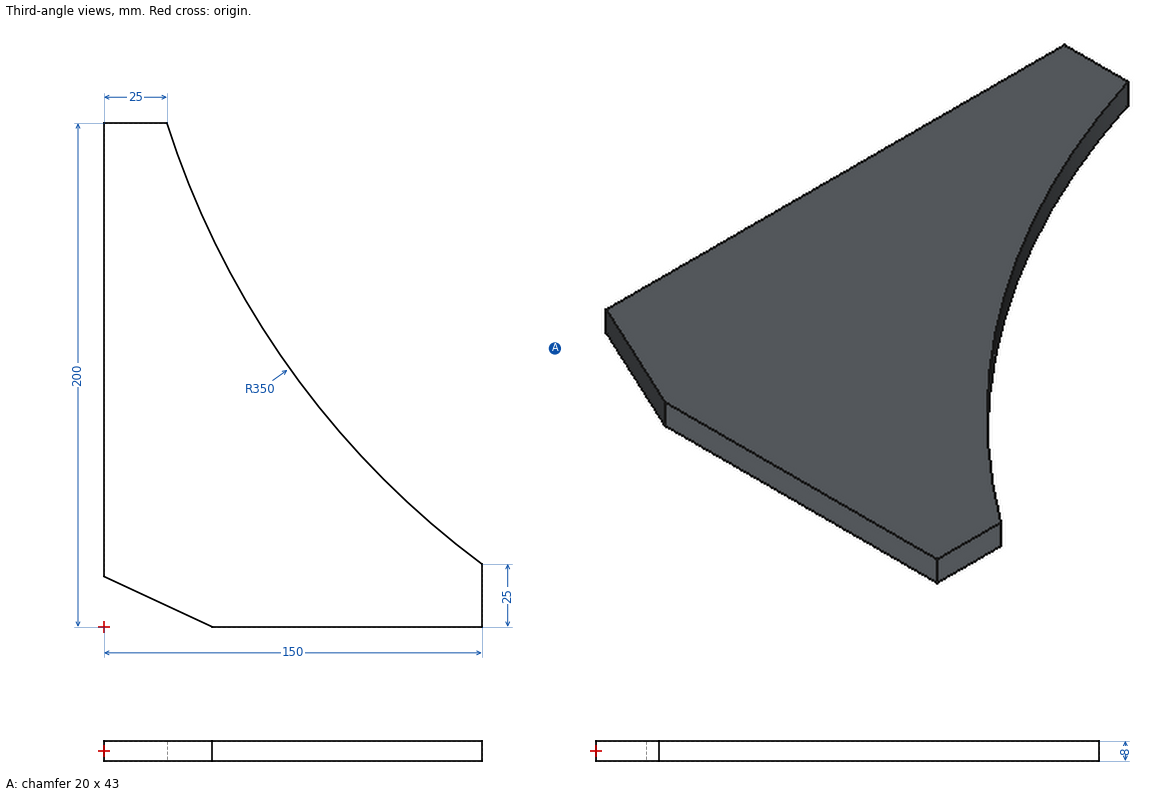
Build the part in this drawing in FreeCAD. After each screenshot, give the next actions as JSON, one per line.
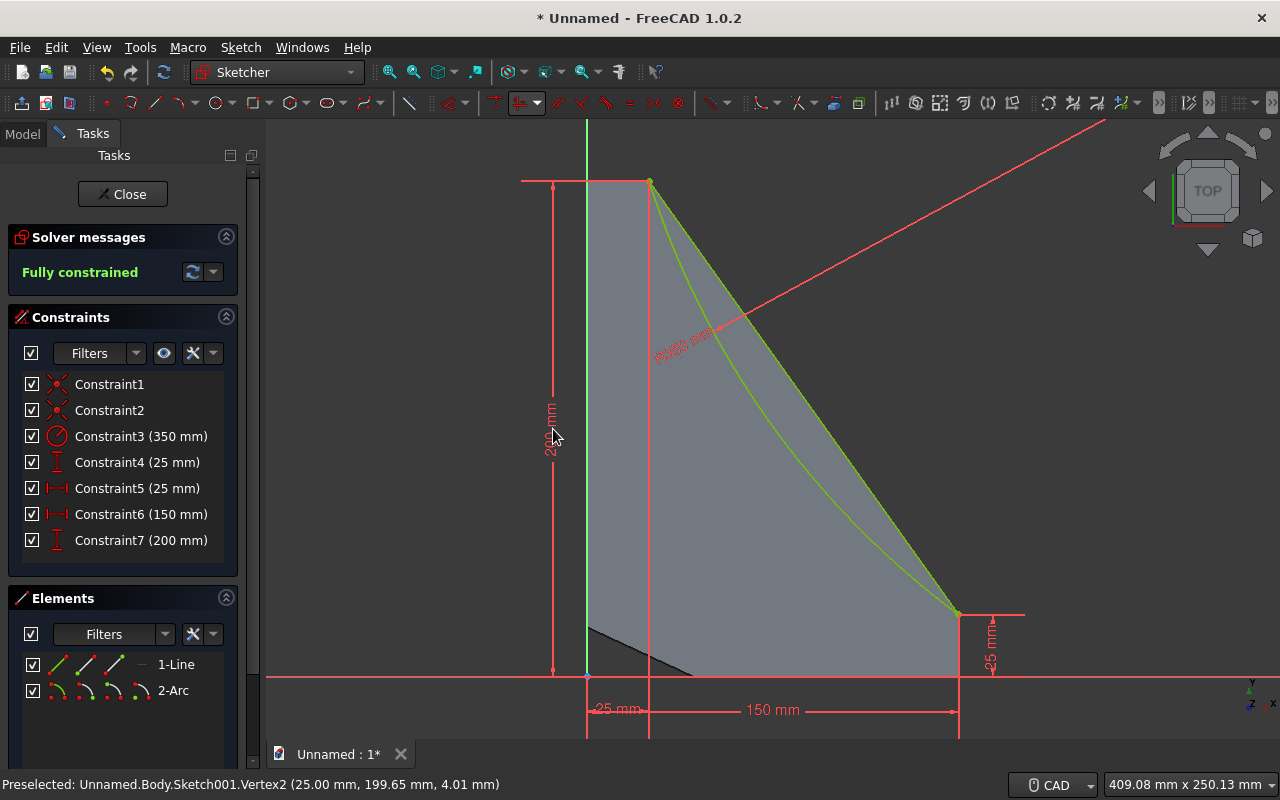
{"action": "left_click", "coordinate": [123, 194]}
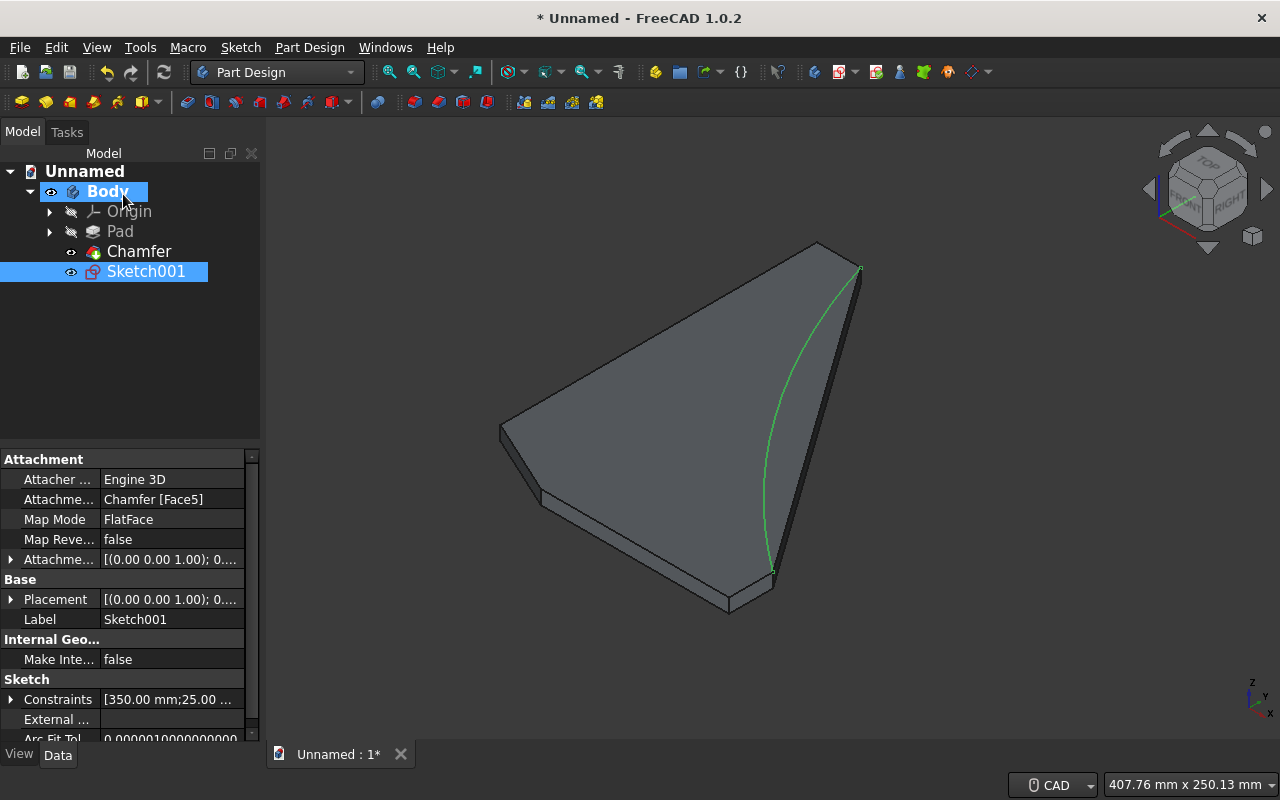
{"action": "left_click", "coordinate": [188, 102]}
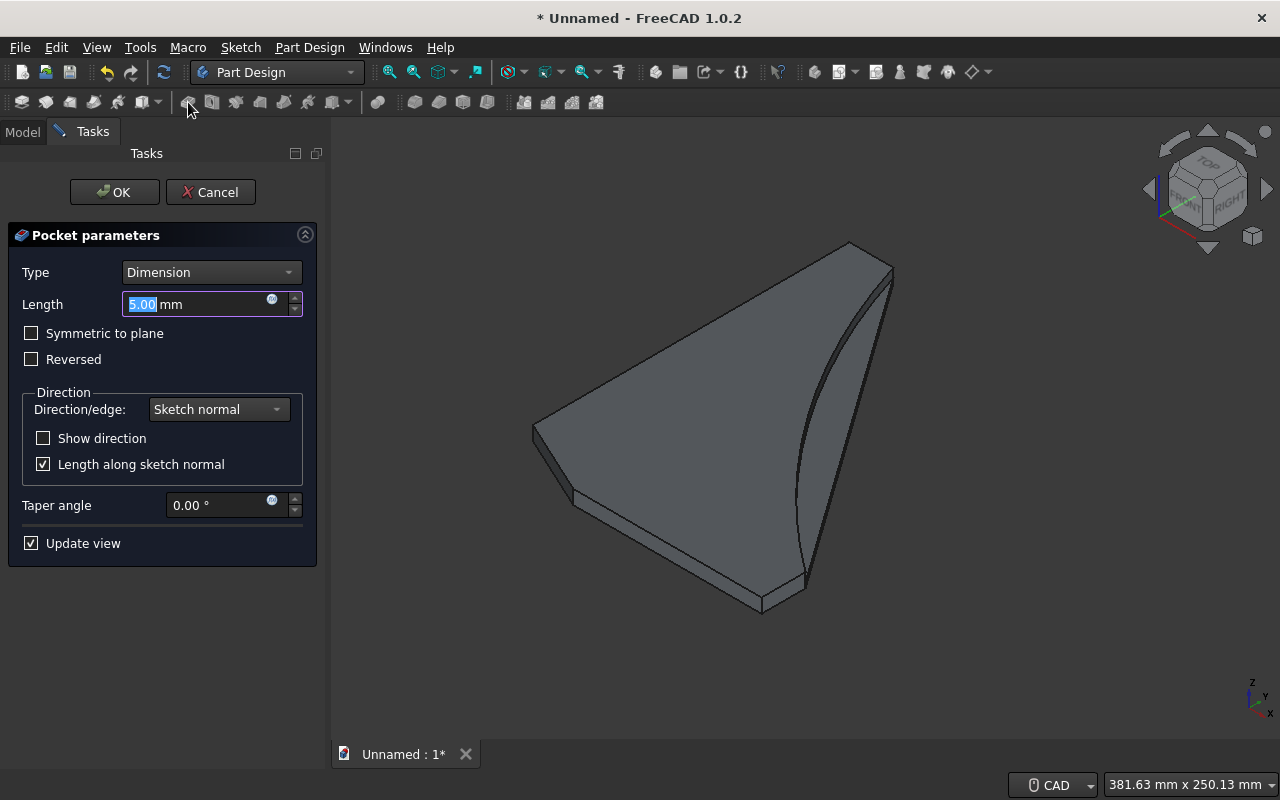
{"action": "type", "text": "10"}
{"action": "key", "text": "Tab"}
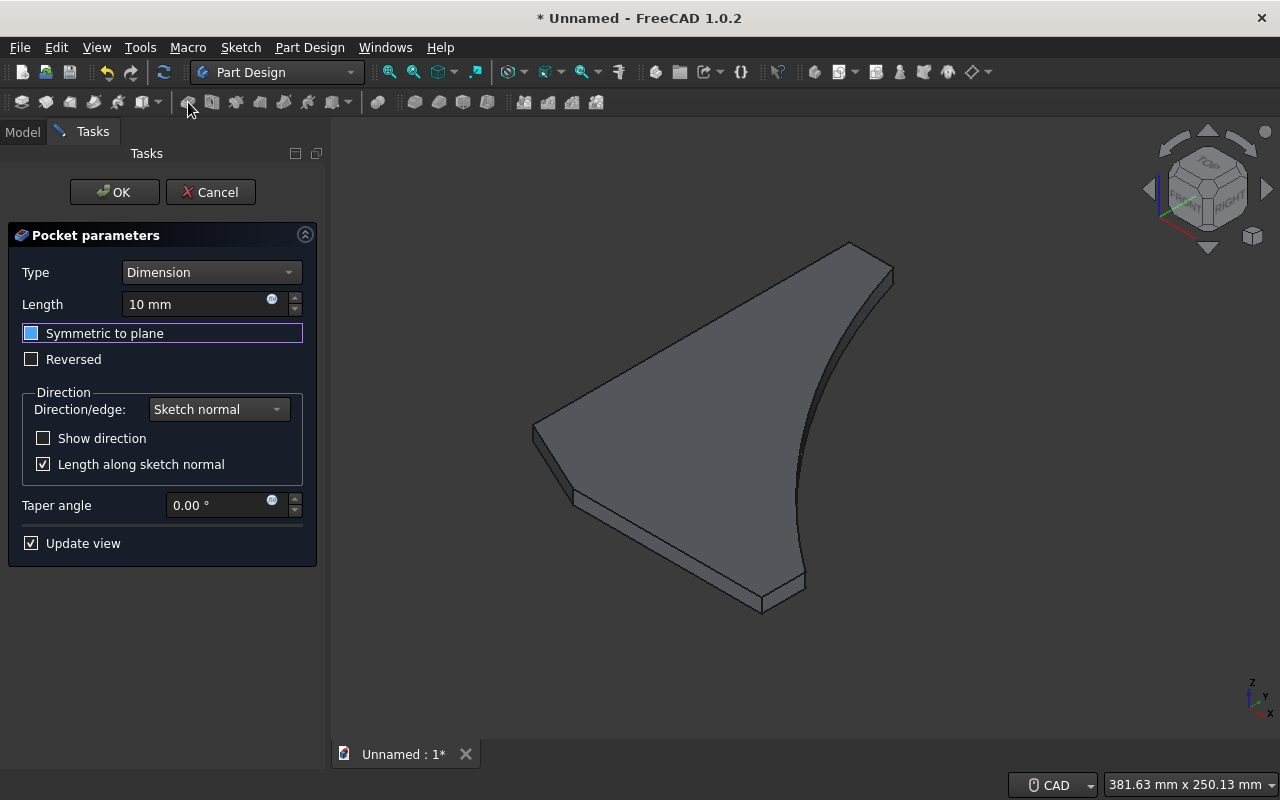
{"action": "left_click", "coordinate": [115, 192]}